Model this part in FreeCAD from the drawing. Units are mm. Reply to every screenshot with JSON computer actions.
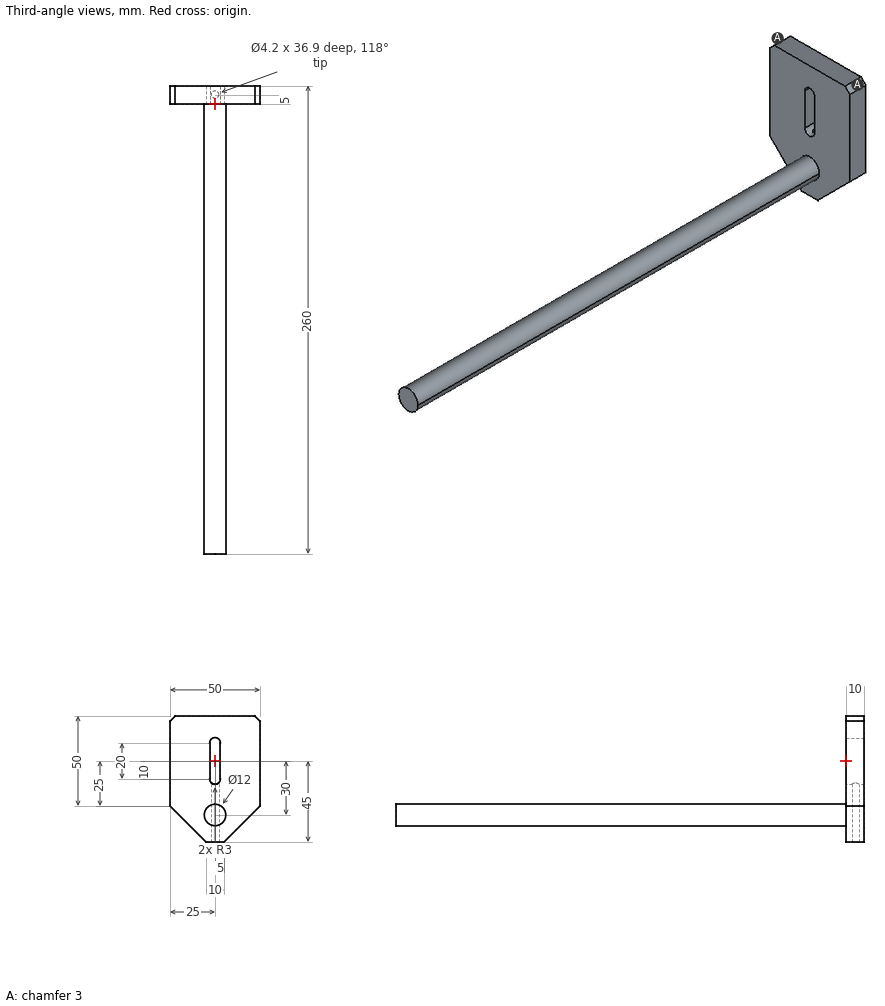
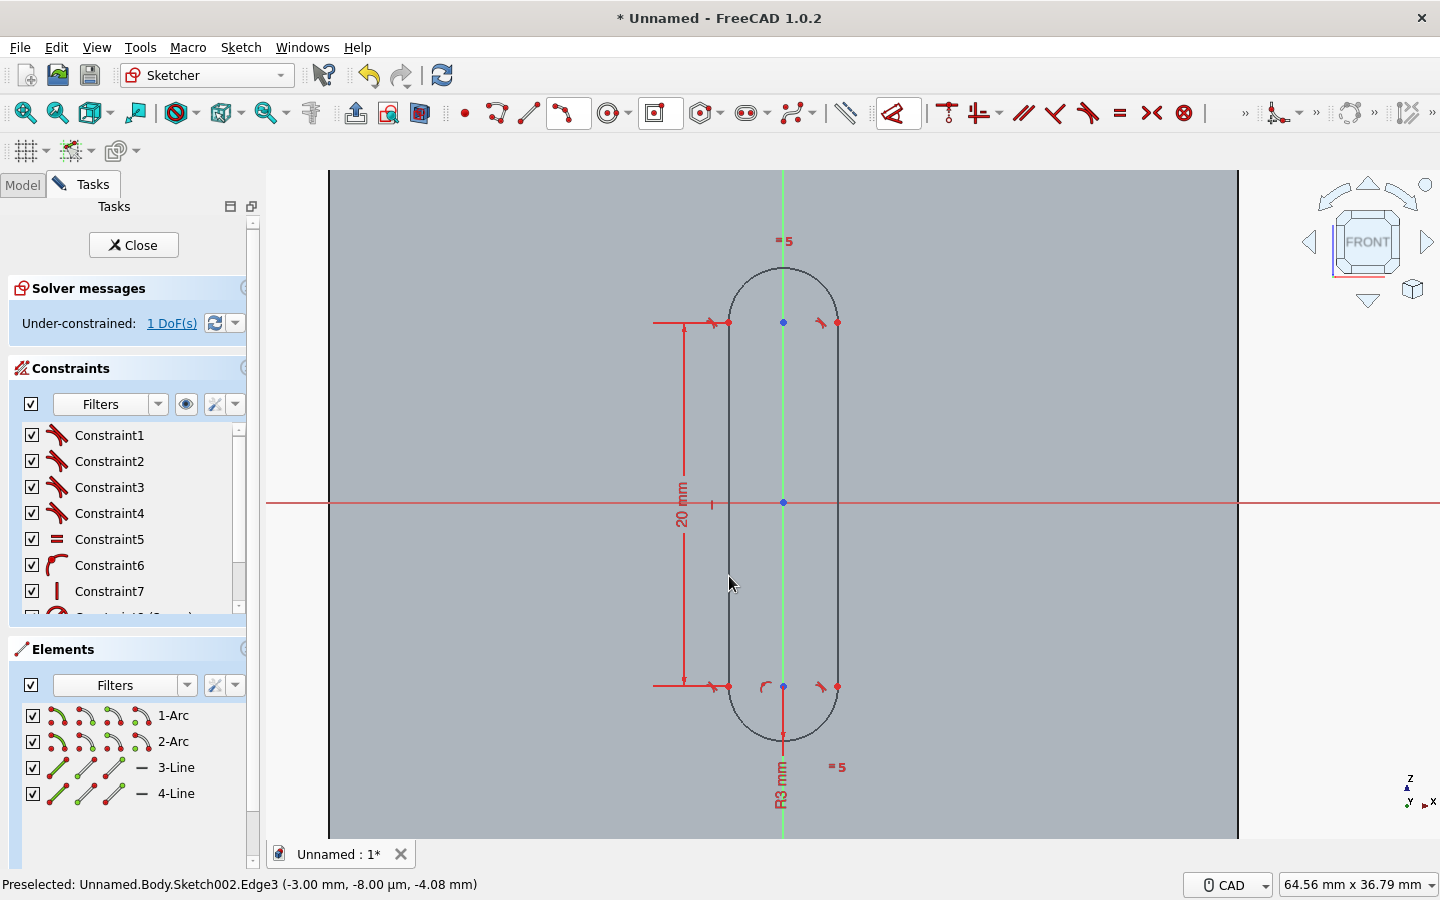
{"action": "left_click", "coordinate": [729, 686]}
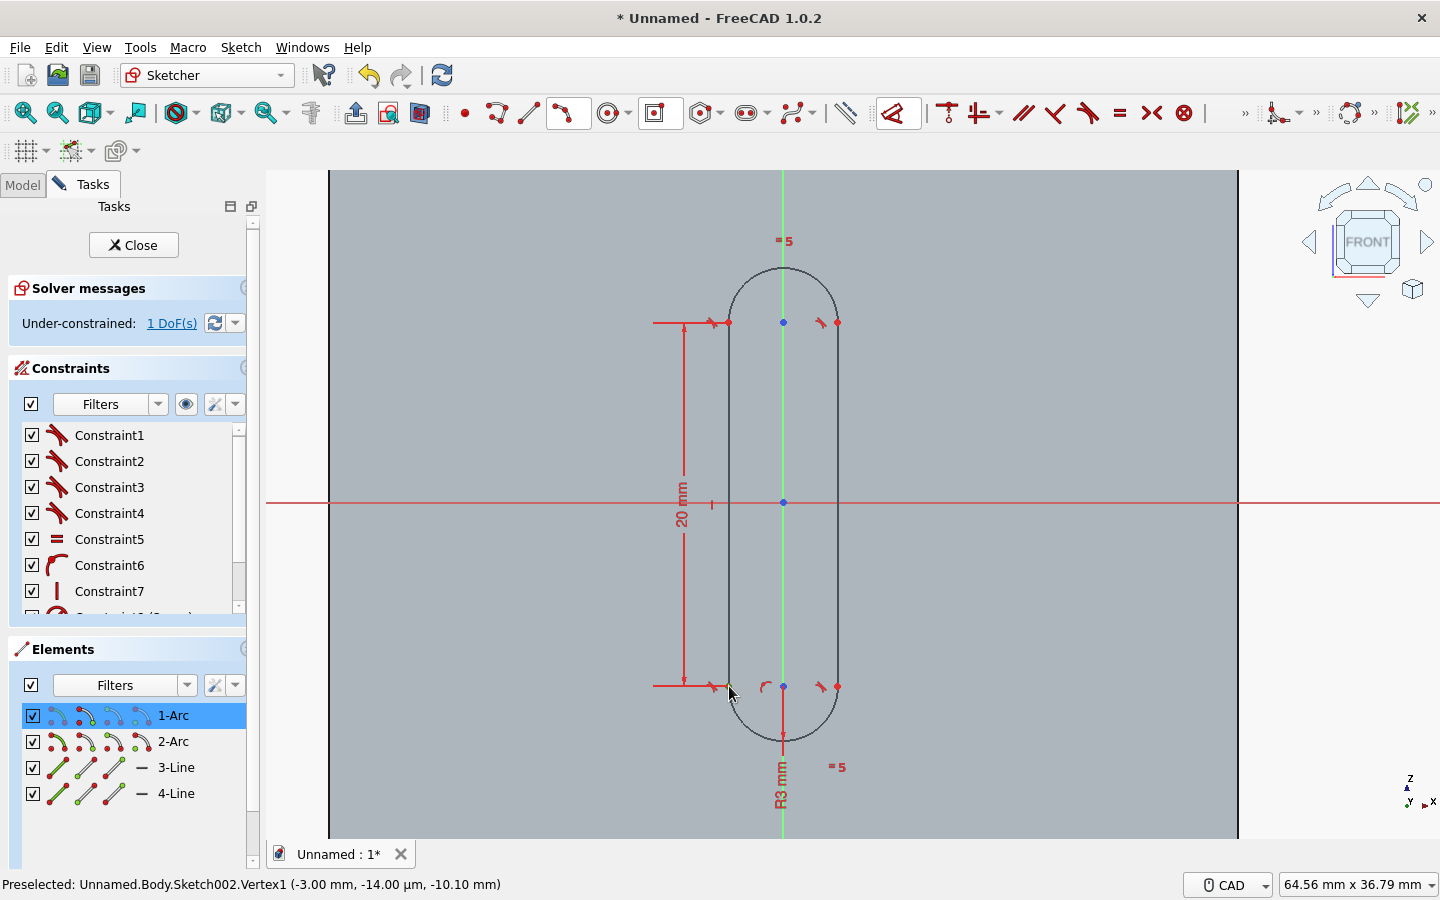
{"action": "left_click", "coordinate": [916, 114]}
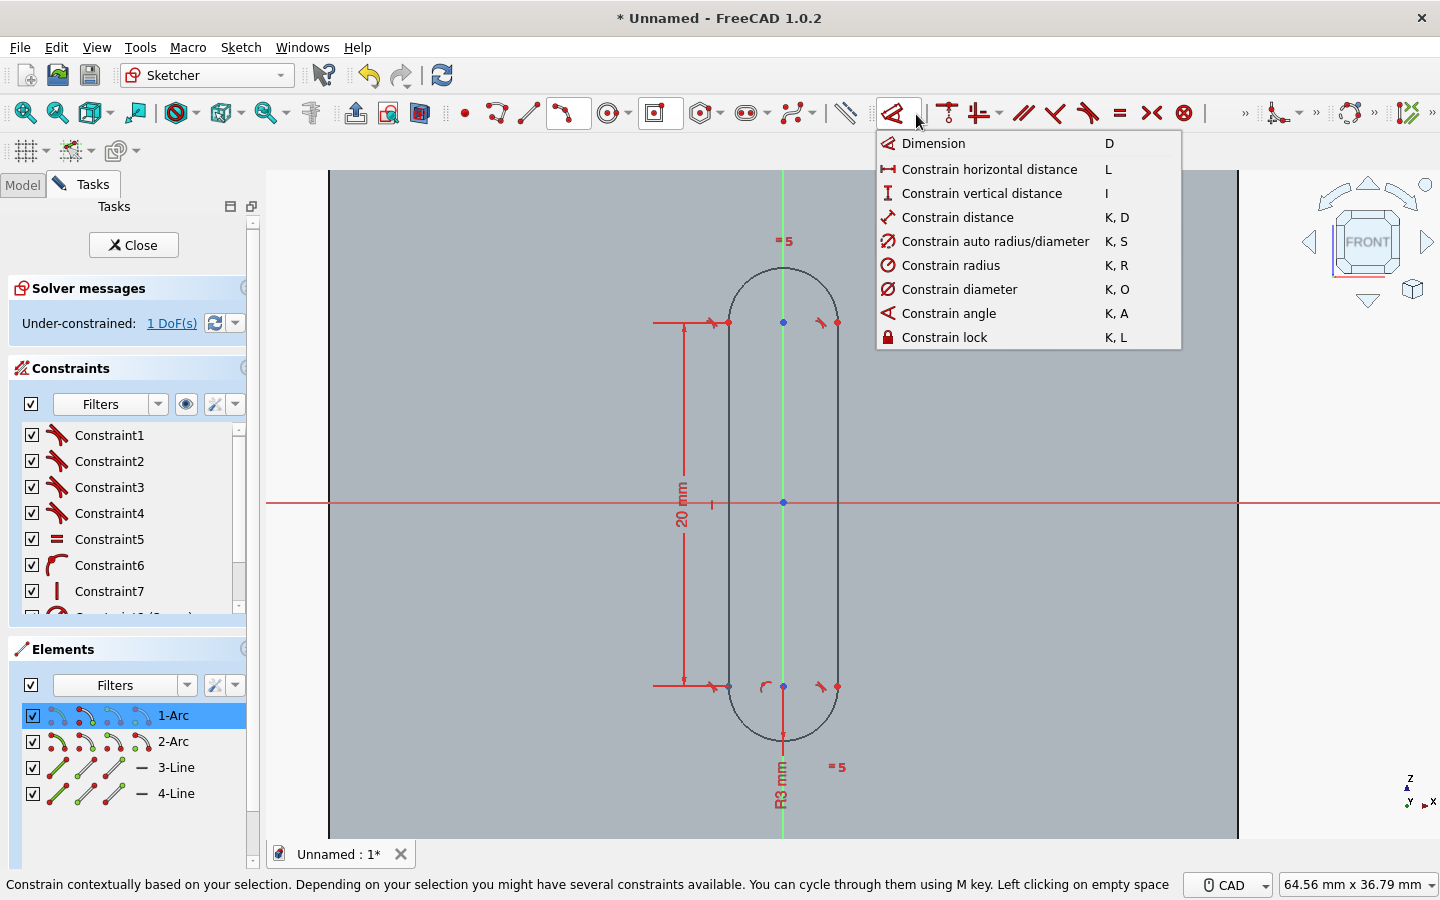
{"action": "left_click", "coordinate": [1029, 193]}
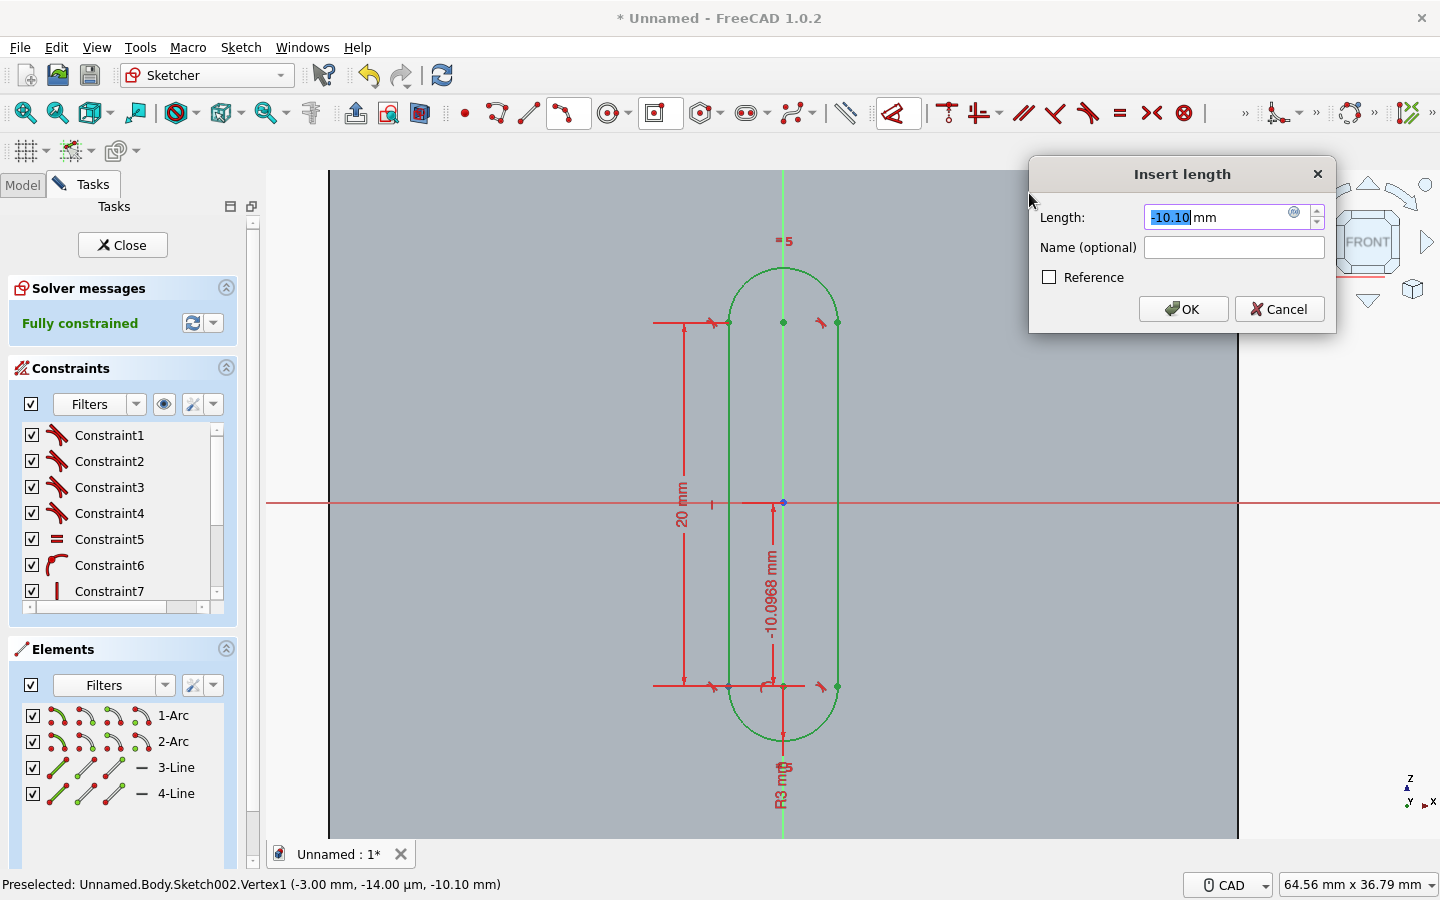
{"action": "type", "text": "-10"}
{"action": "key", "text": "Return"}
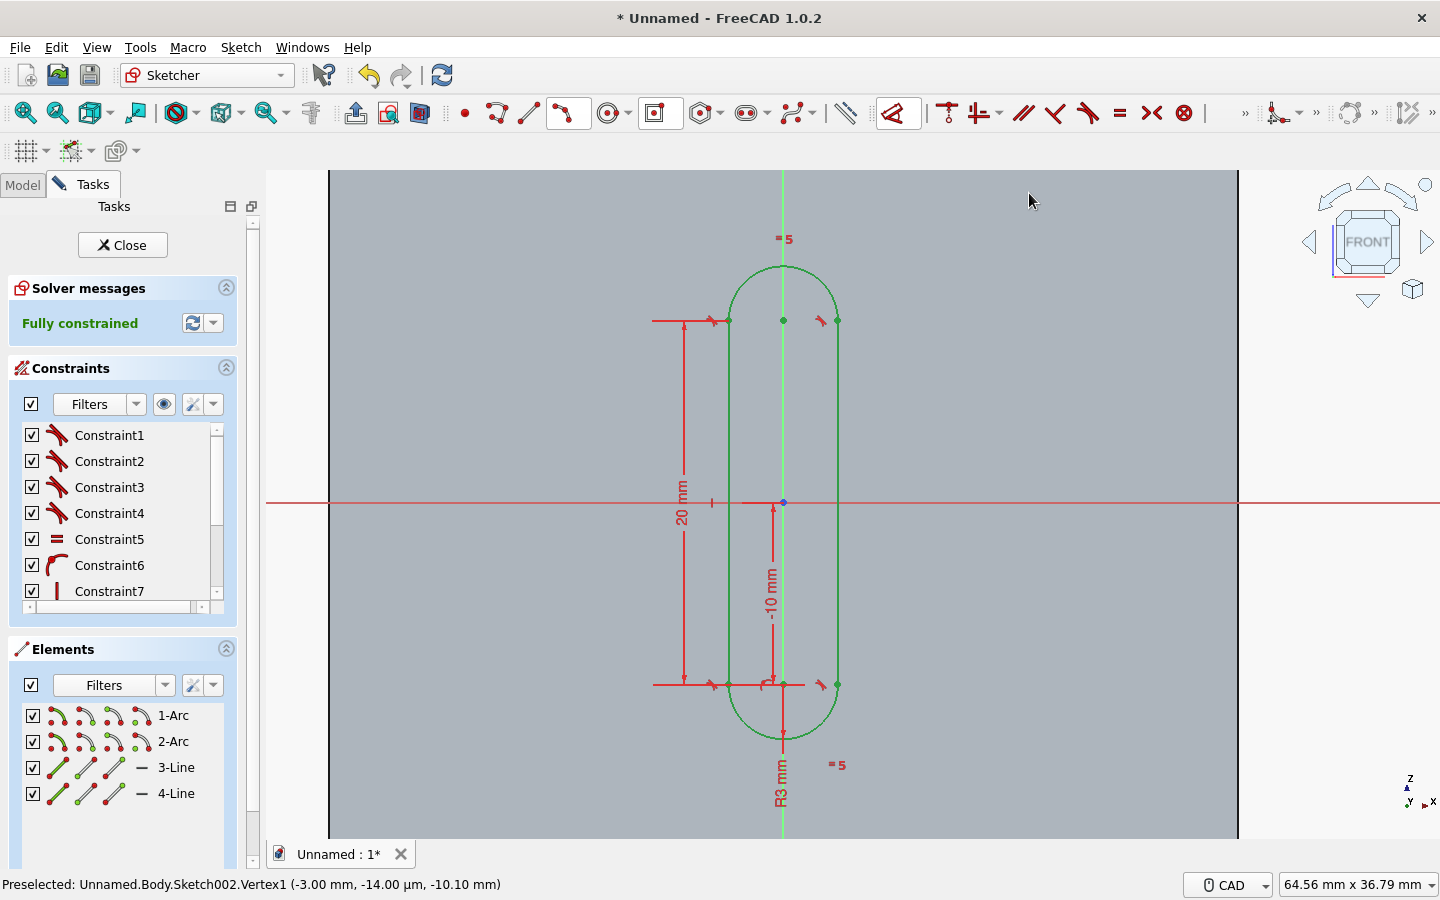
{"action": "left_click", "coordinate": [123, 245]}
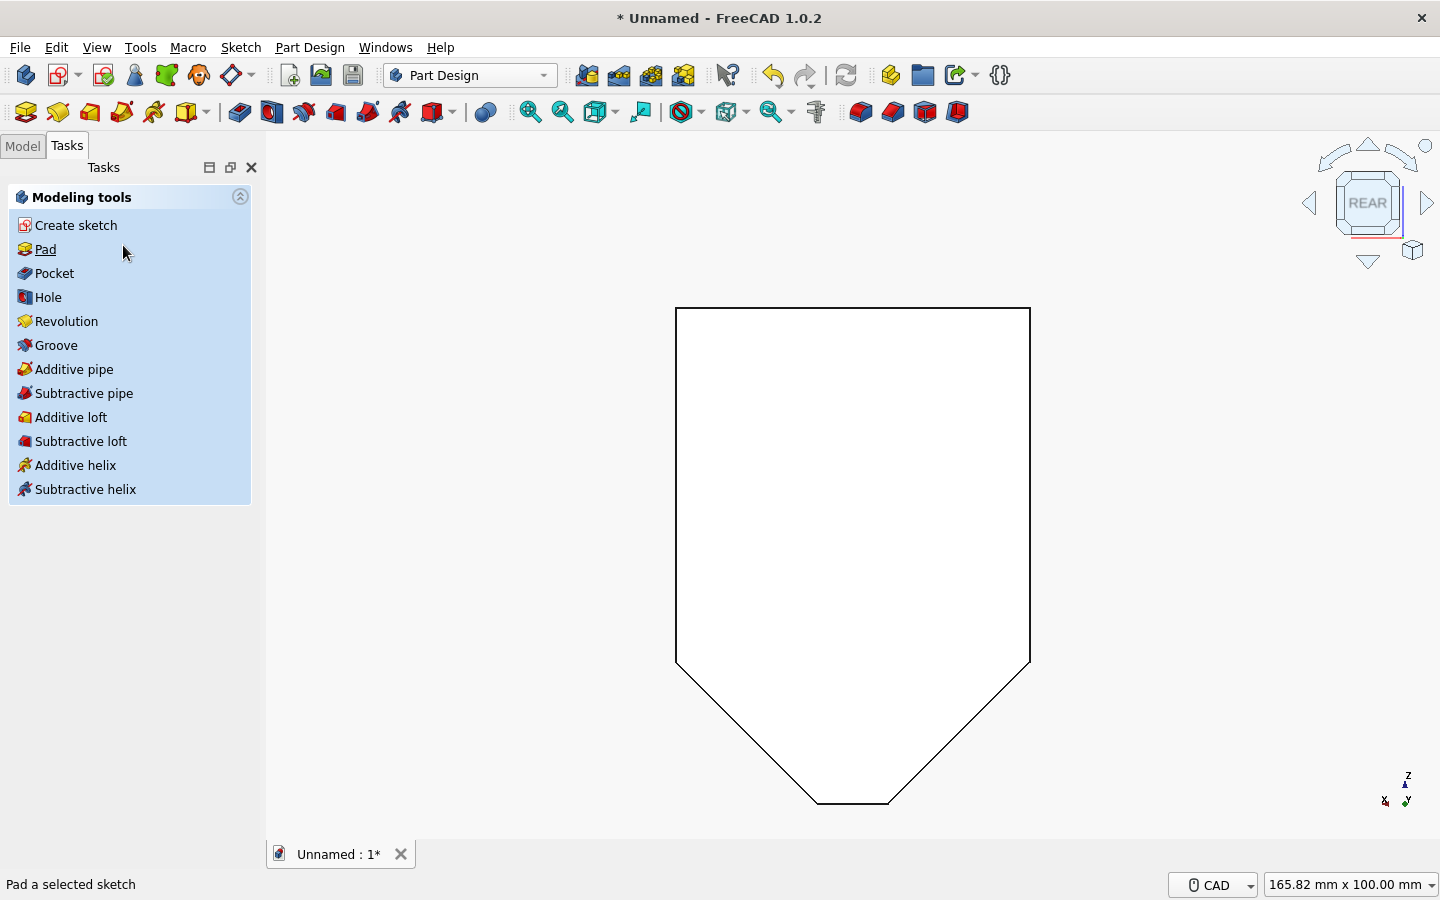
{"action": "left_click", "coordinate": [240, 112]}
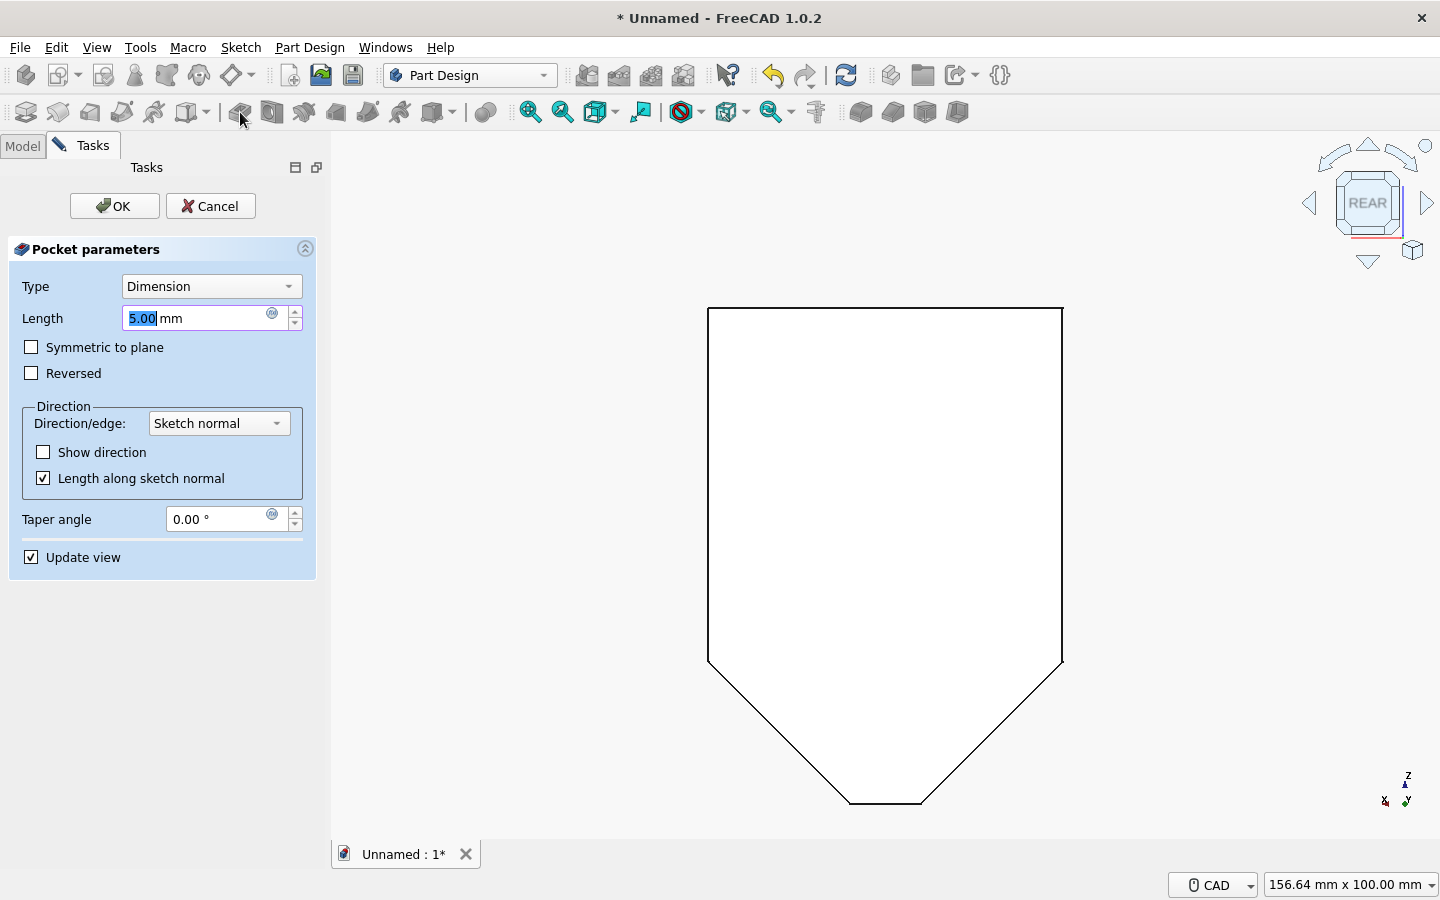
{"action": "left_click", "coordinate": [212, 286]}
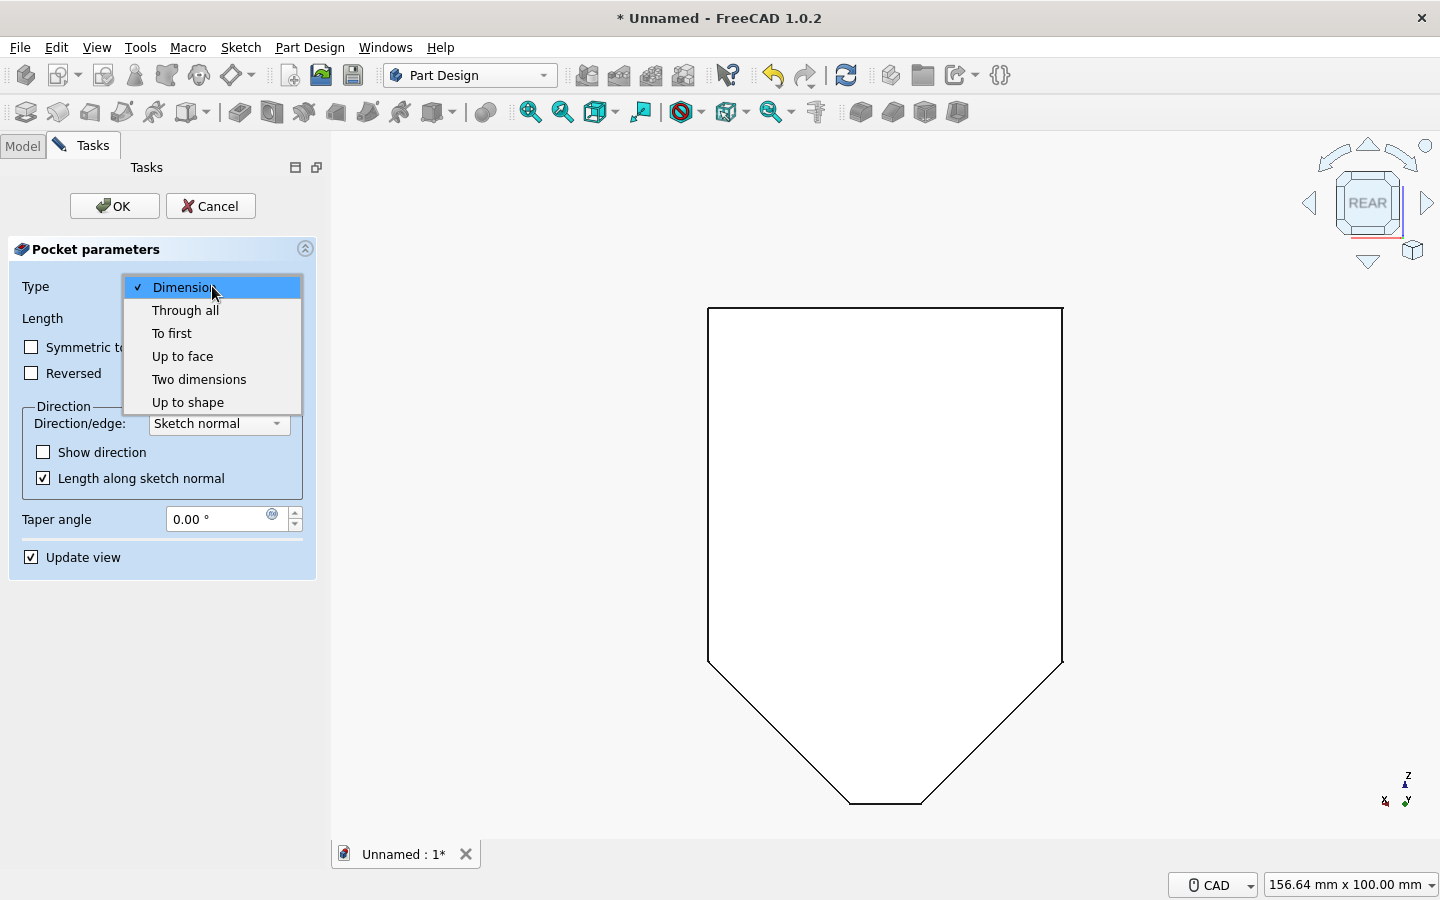
{"action": "left_click", "coordinate": [212, 310]}